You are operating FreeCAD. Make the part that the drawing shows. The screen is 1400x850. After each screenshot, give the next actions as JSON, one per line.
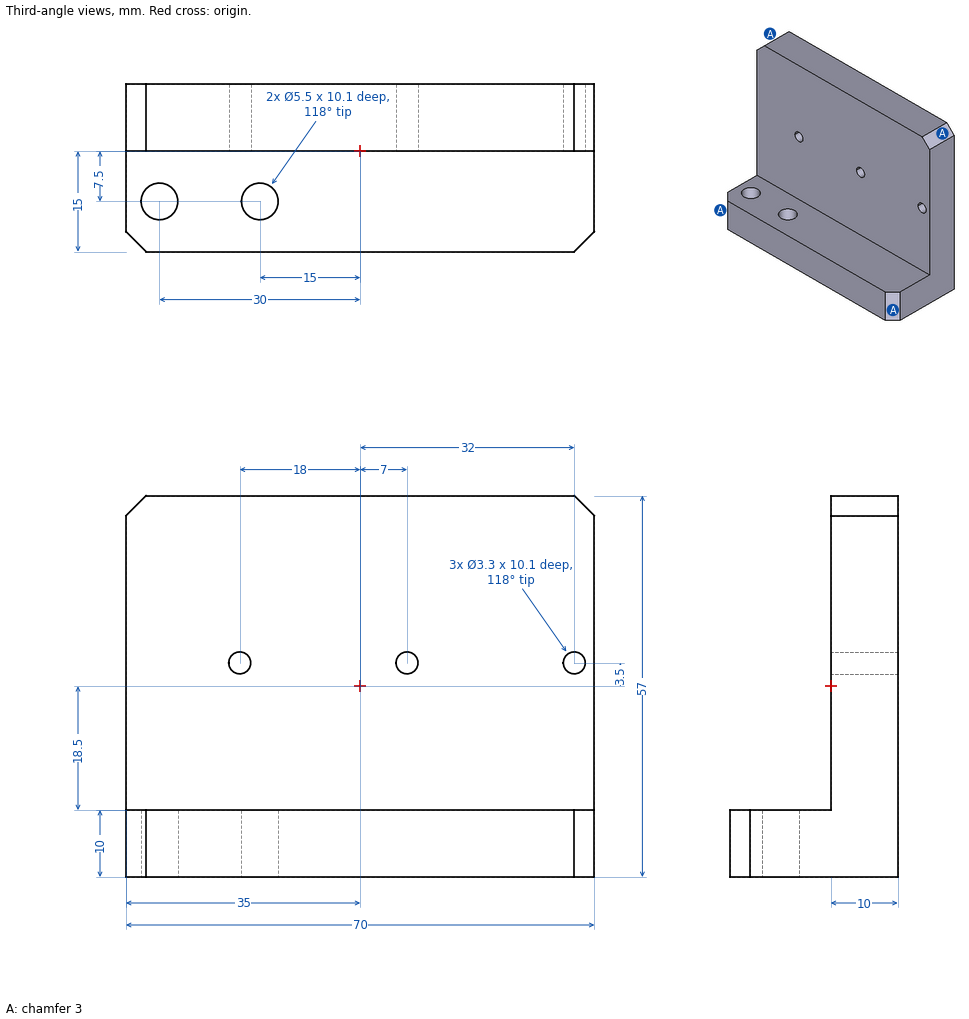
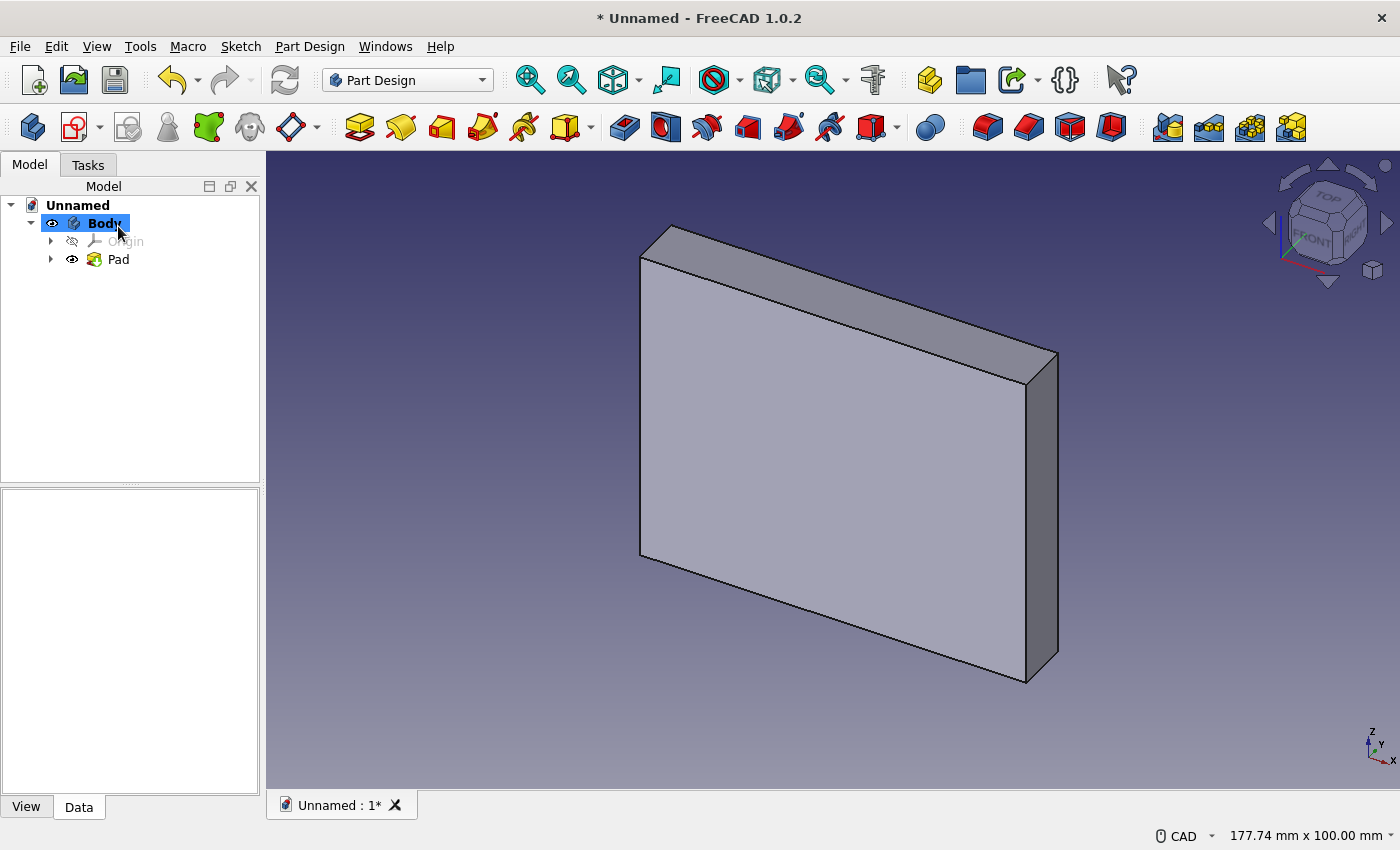
{"action": "left_click", "coordinate": [833, 469]}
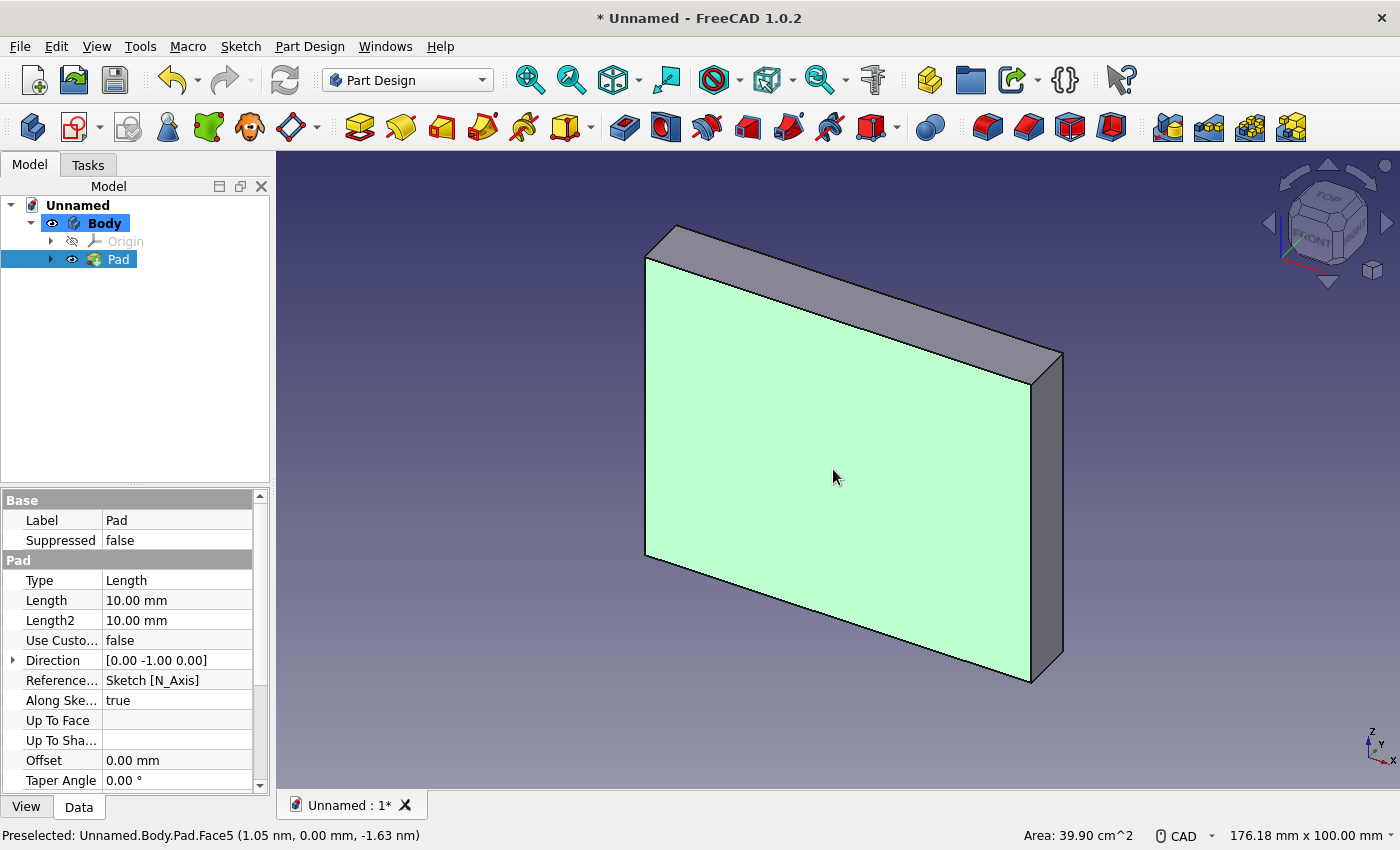
{"action": "left_click", "coordinate": [74, 128]}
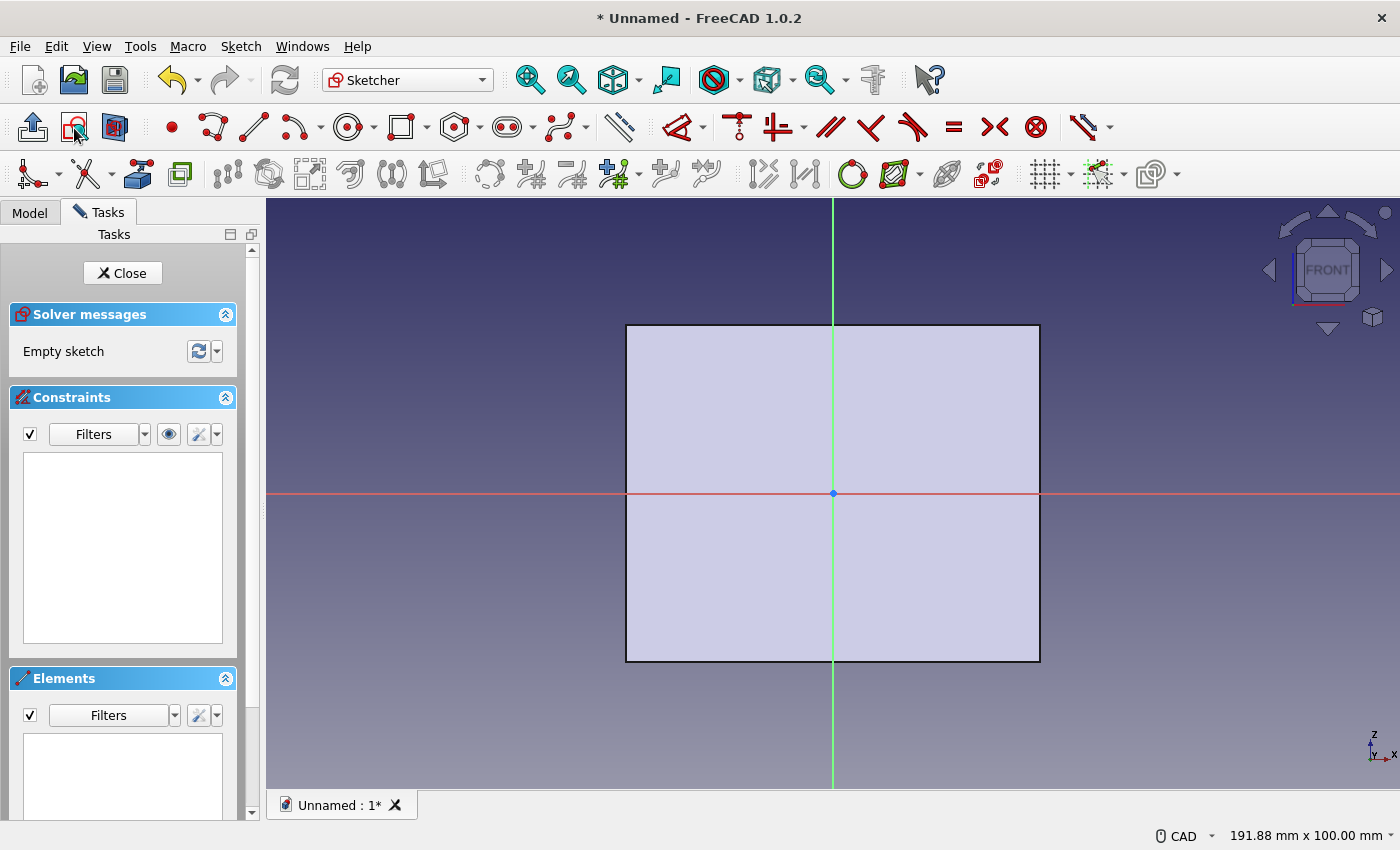
{"action": "scroll", "coordinate": [972, 749], "scroll_direction": "up", "scroll_amount": 2}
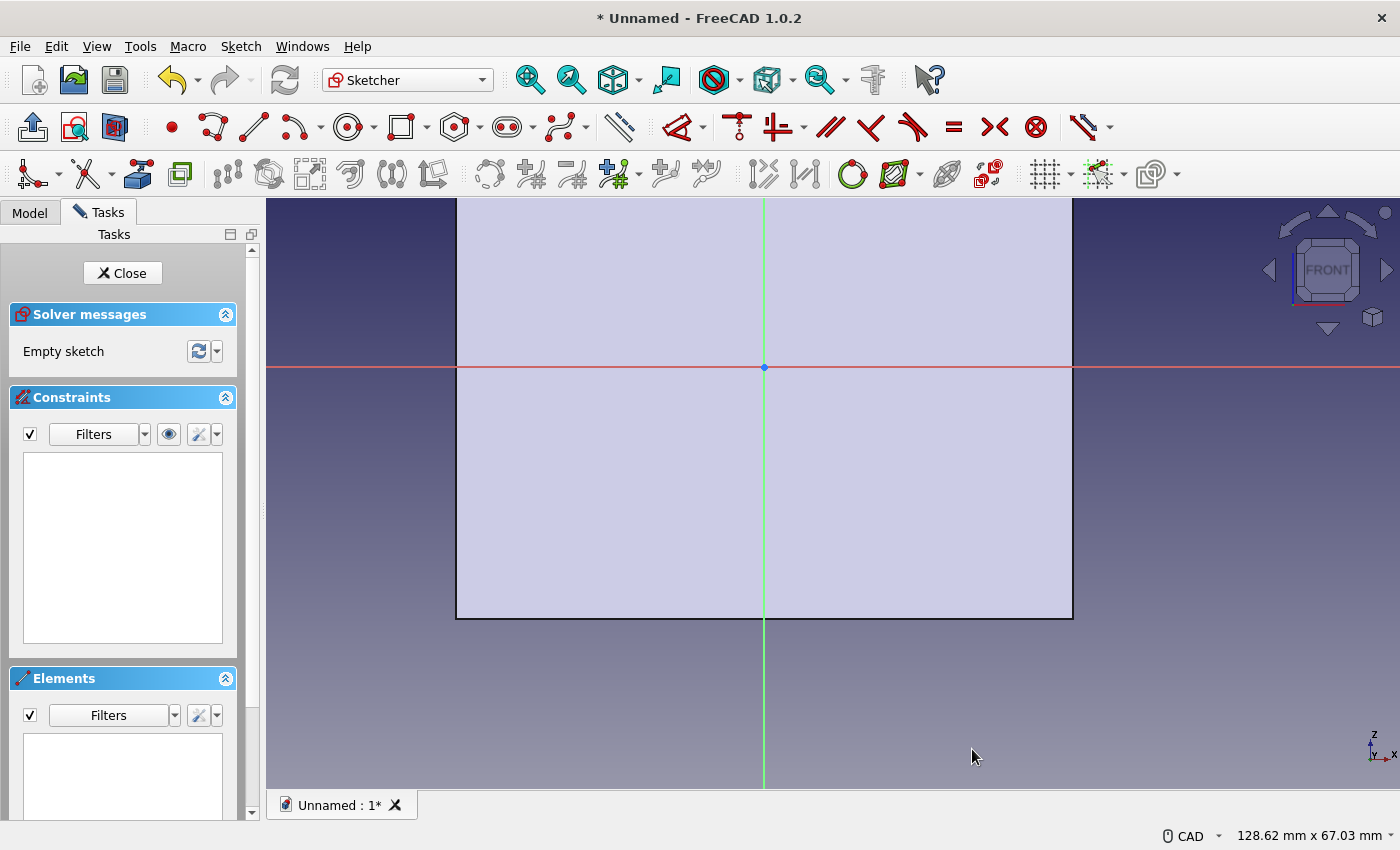
{"action": "left_click", "coordinate": [400, 128]}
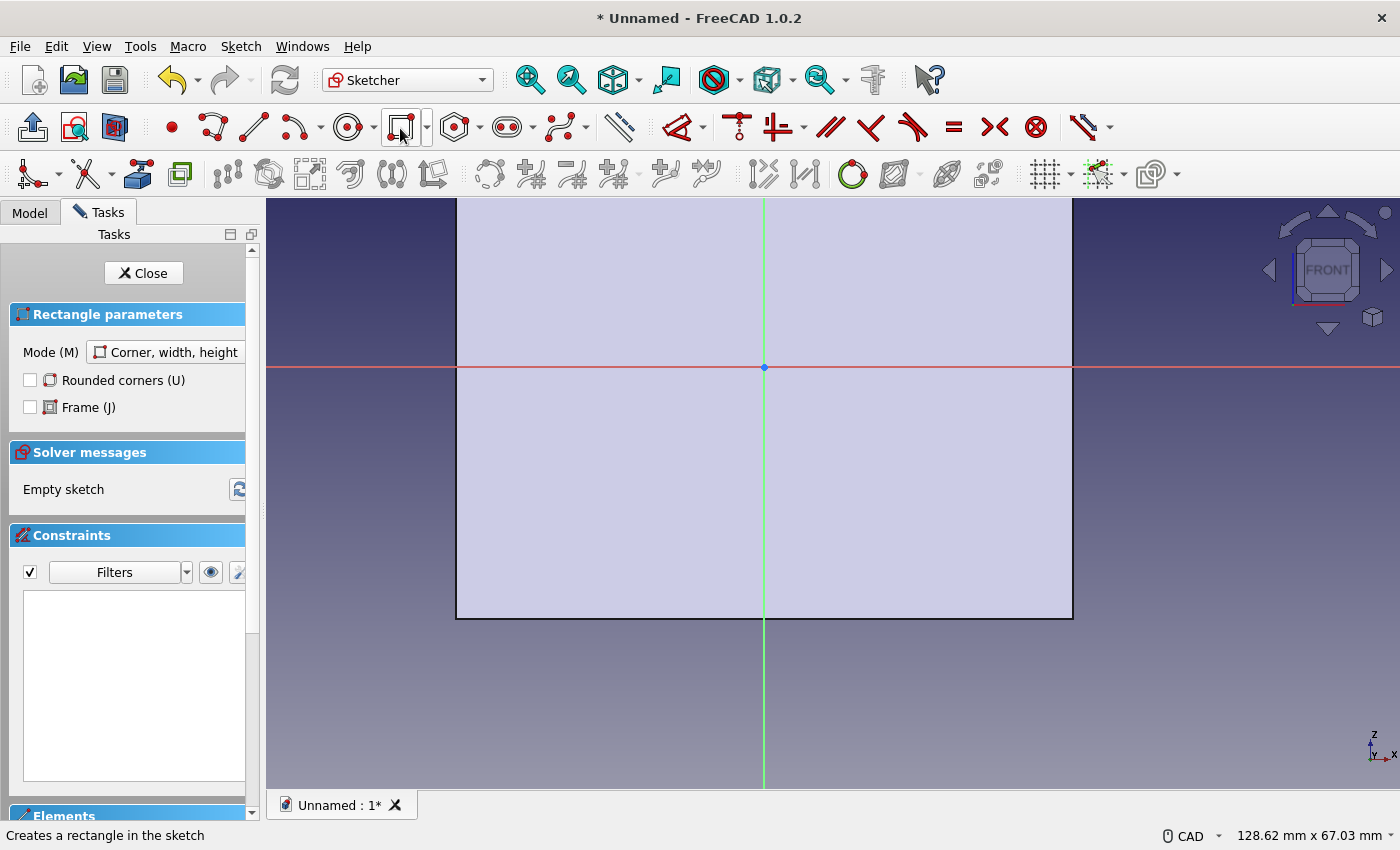
{"action": "left_click", "coordinate": [456, 530]}
{"action": "left_click", "coordinate": [1073, 619]}
{"action": "key", "text": "Escape"}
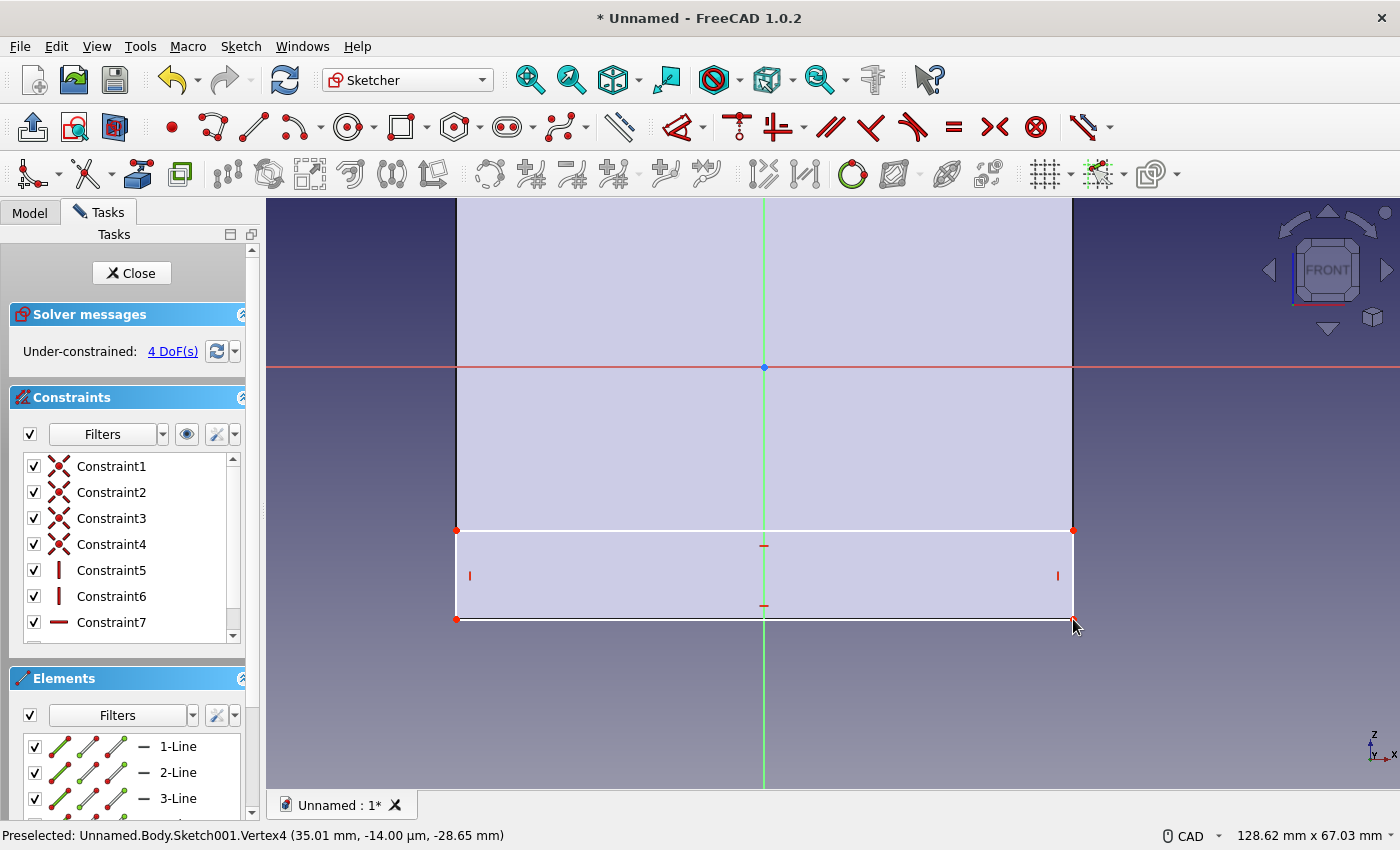
{"action": "left_click", "coordinate": [676, 128]}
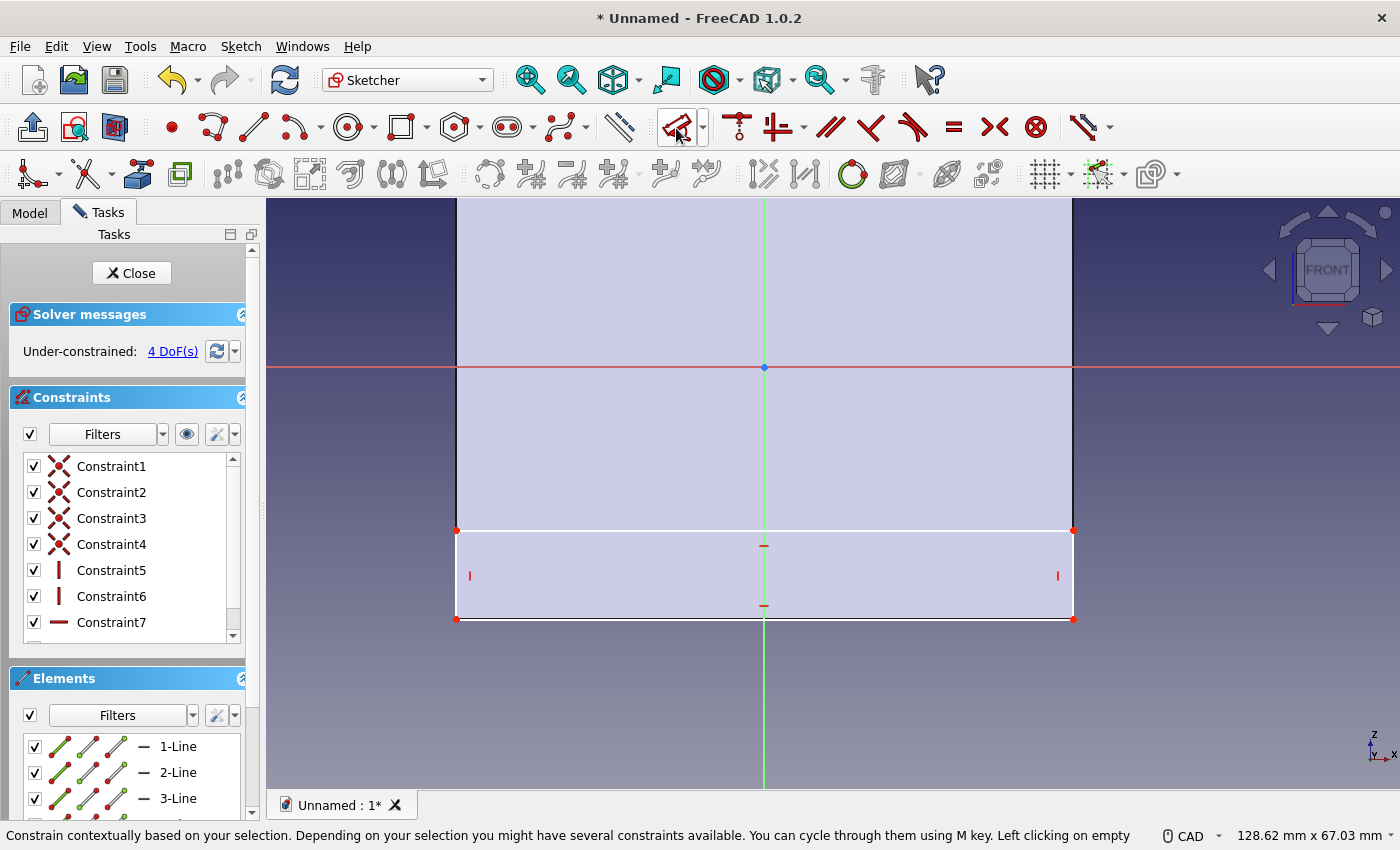
{"action": "left_click", "coordinate": [456, 558]}
{"action": "left_click", "coordinate": [422, 576]}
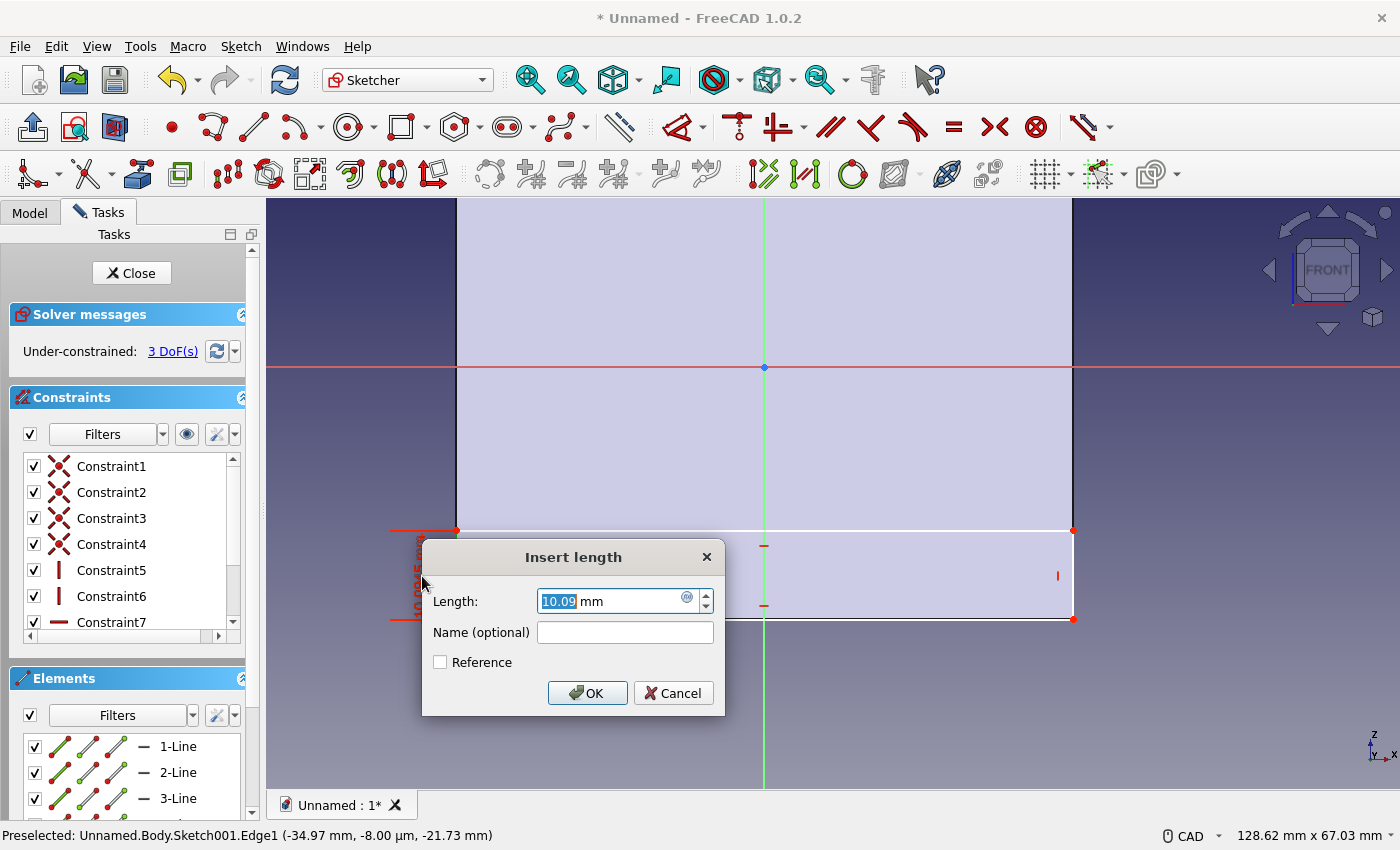
{"action": "type", "text": "10"}
{"action": "key", "text": "Return"}